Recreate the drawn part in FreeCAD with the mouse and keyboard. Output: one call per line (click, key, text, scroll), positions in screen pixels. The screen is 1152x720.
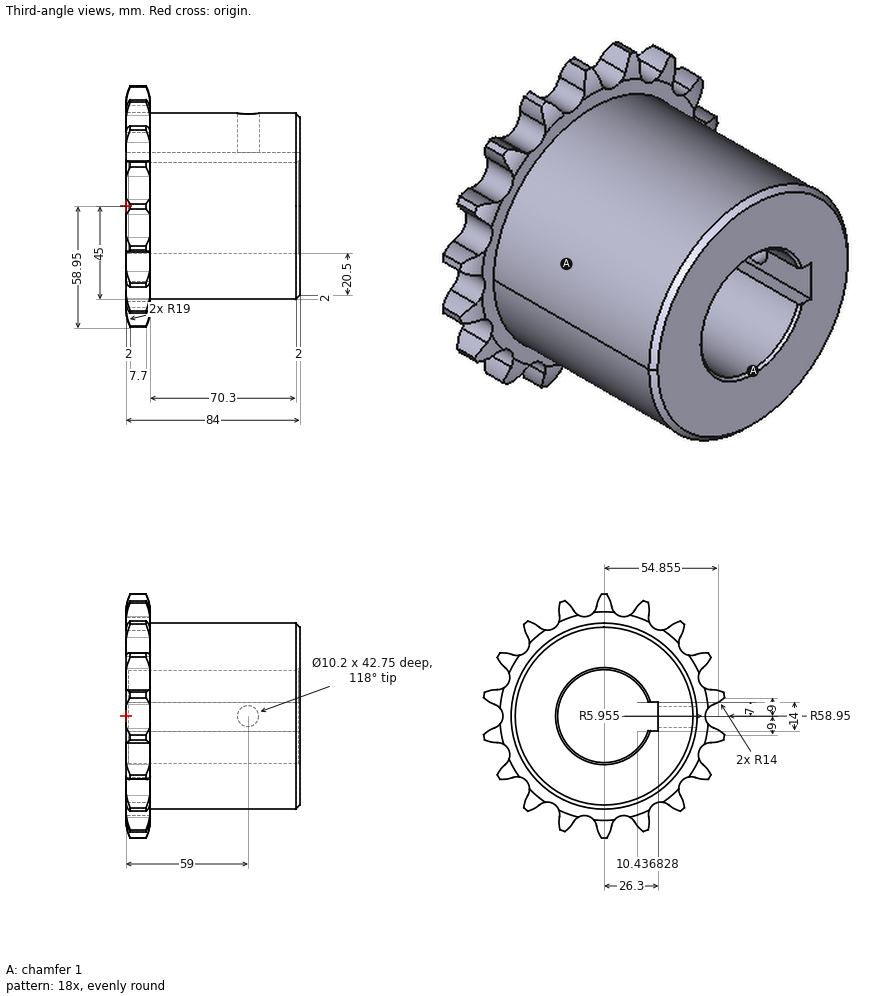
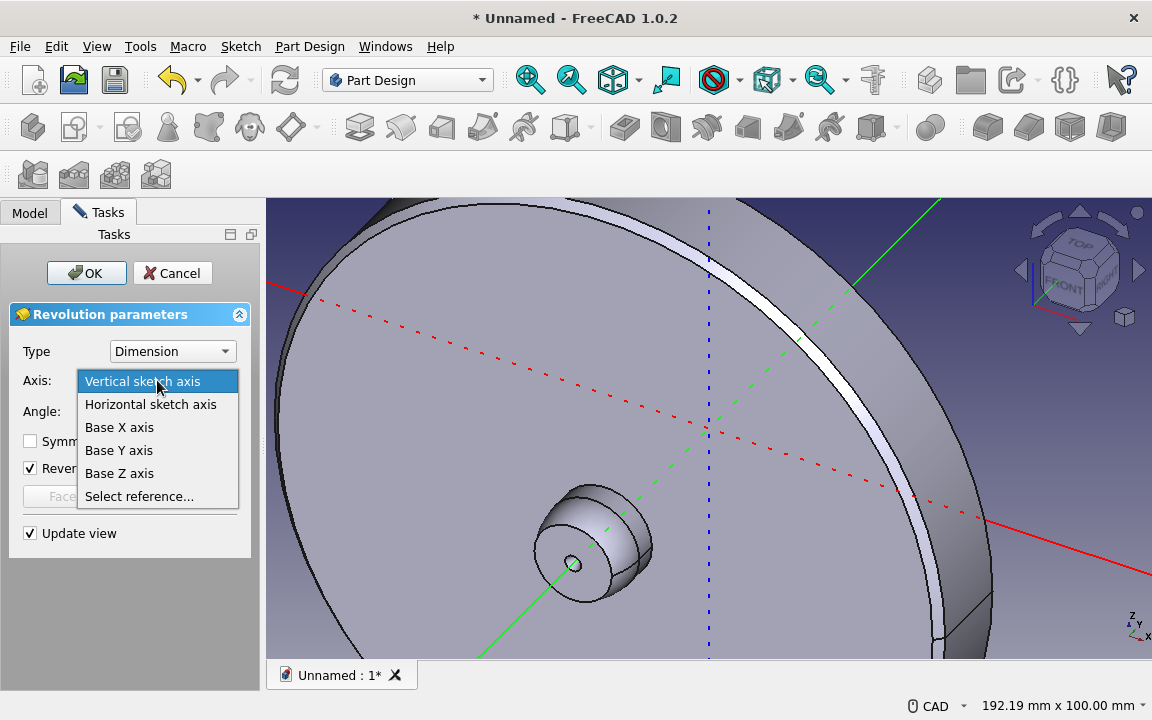
click(156, 404)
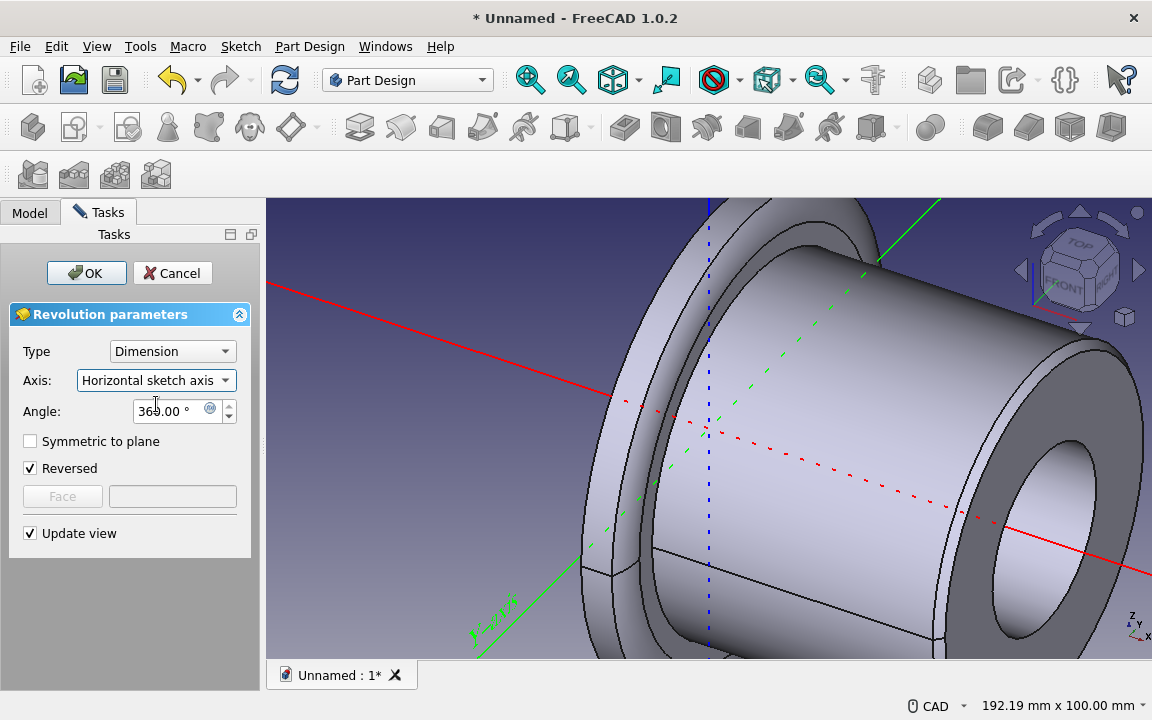
click(87, 273)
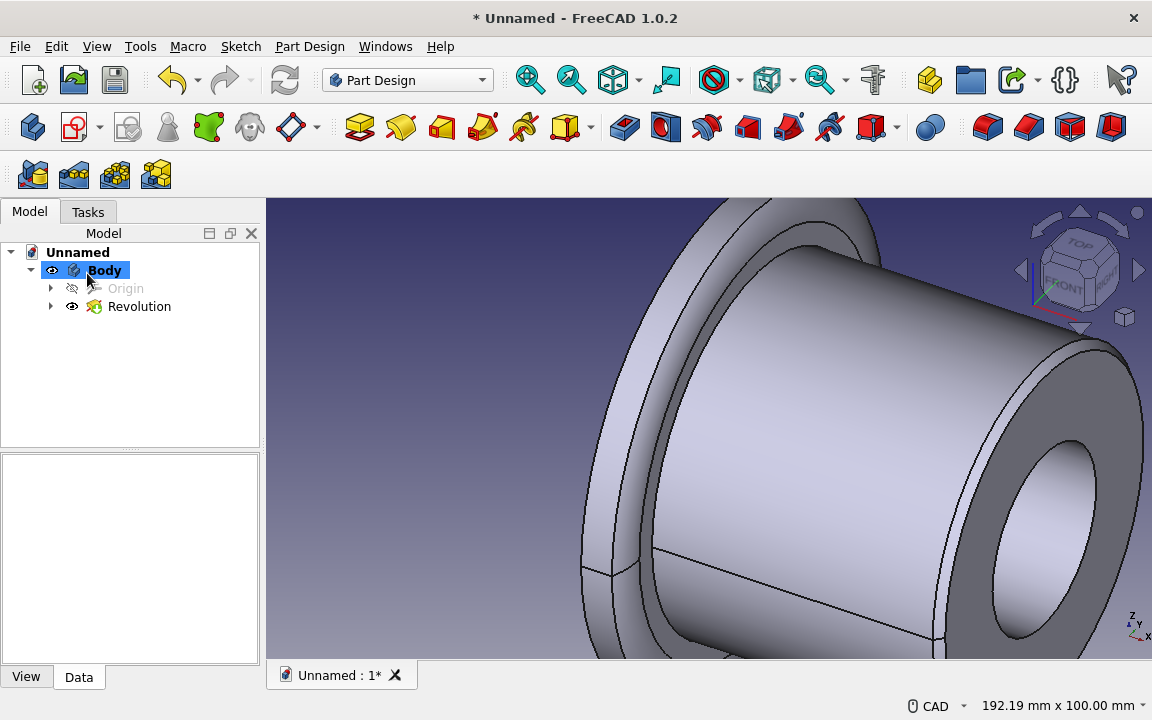
click(531, 80)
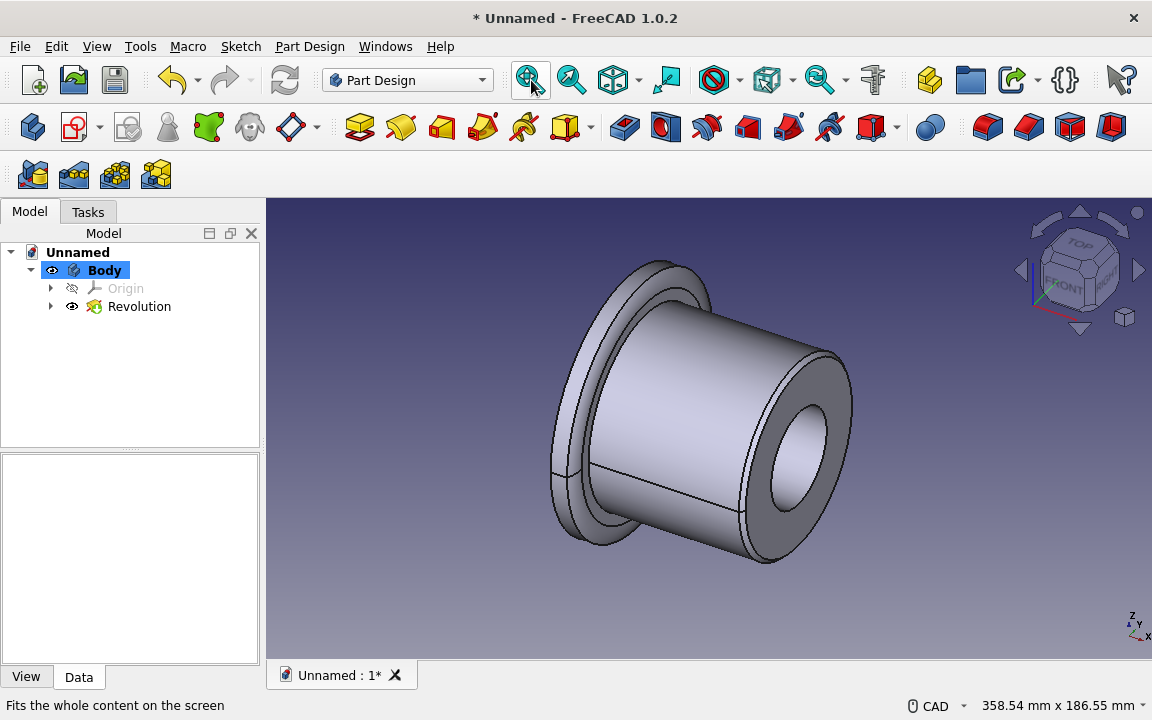
click(827, 430)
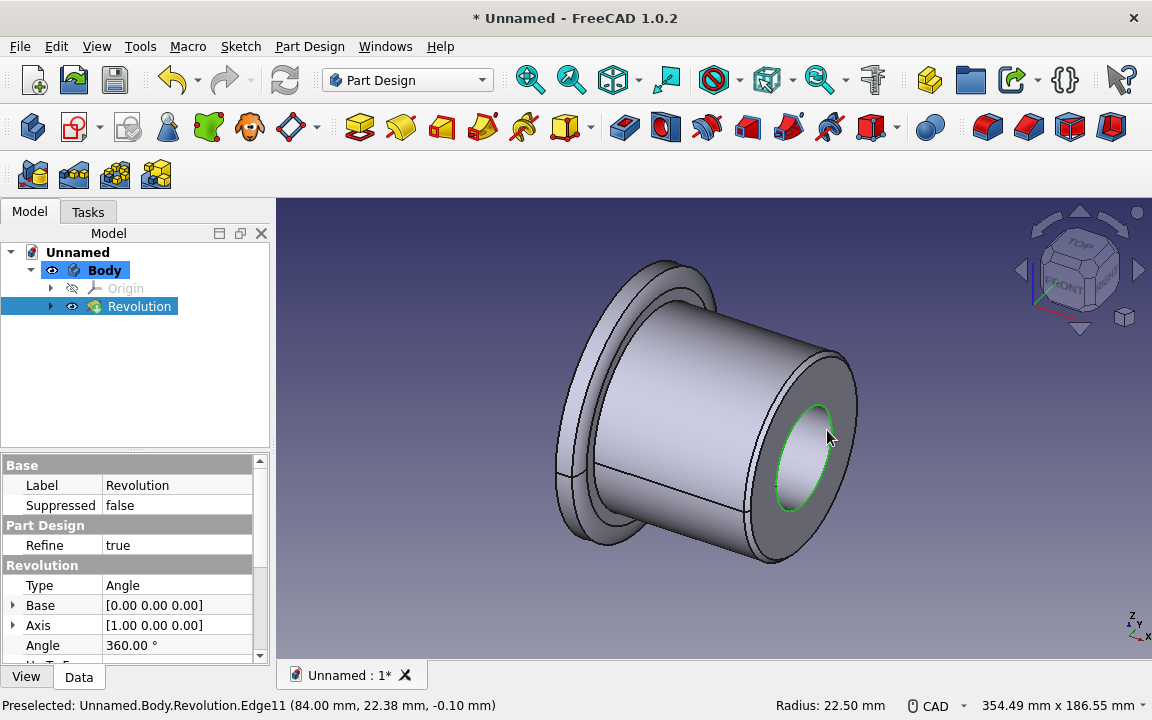
key(0)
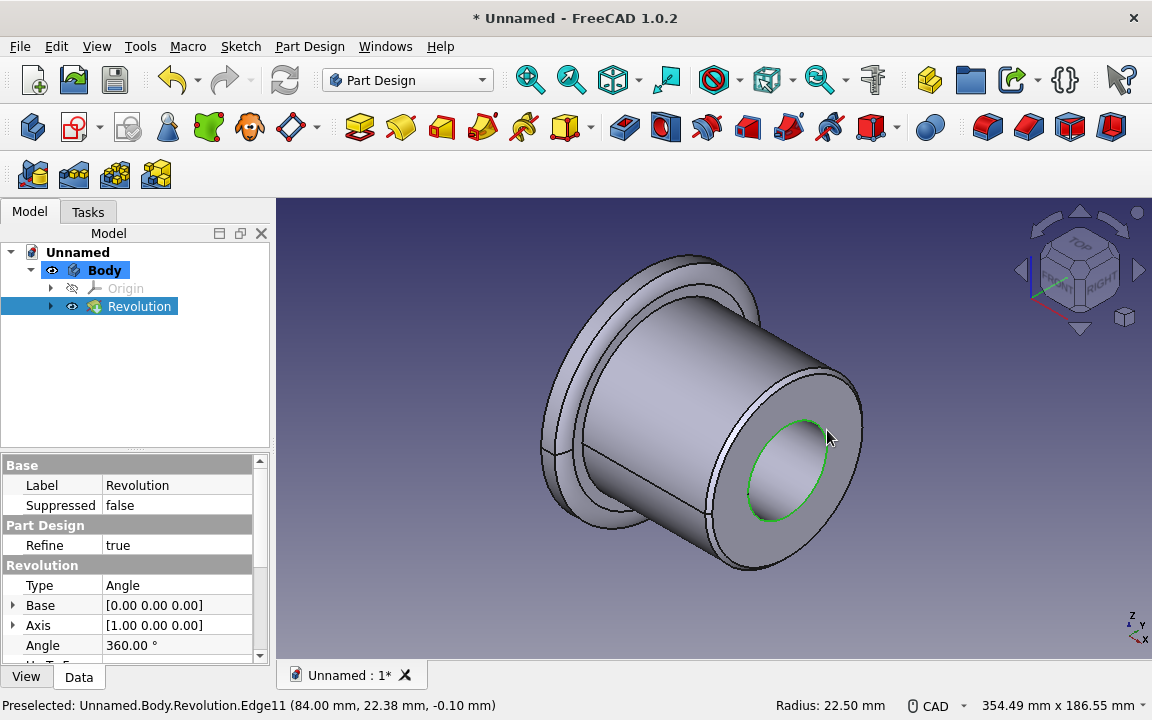
key(2)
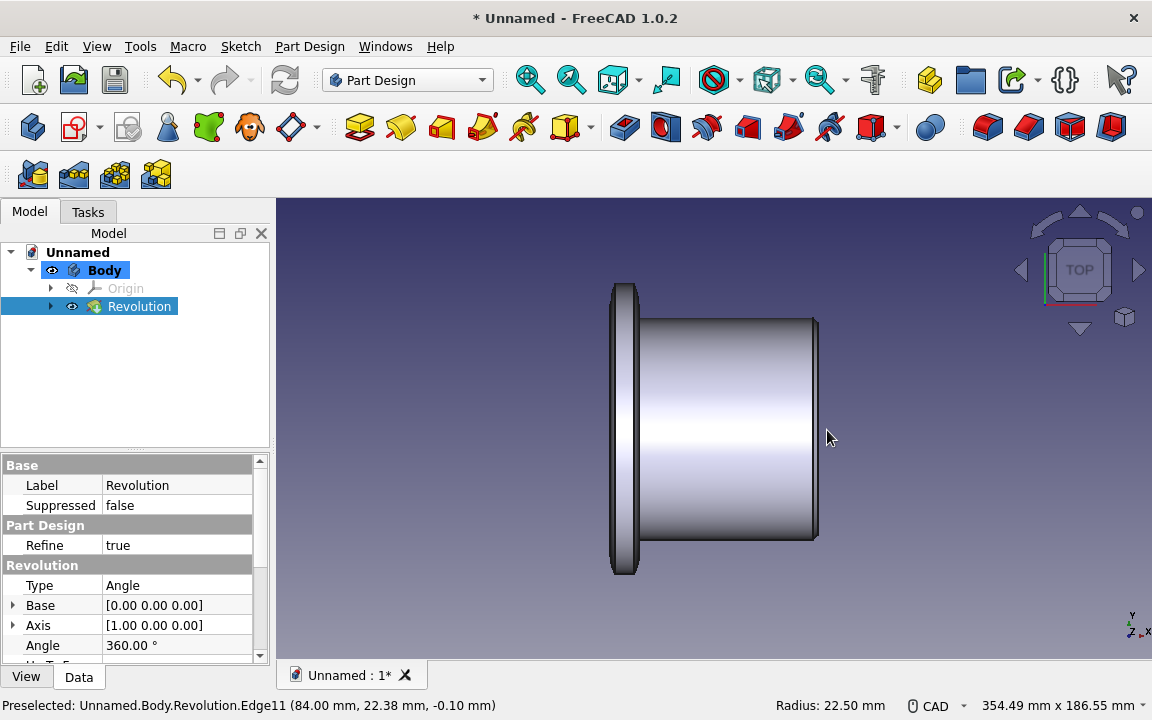
key(1)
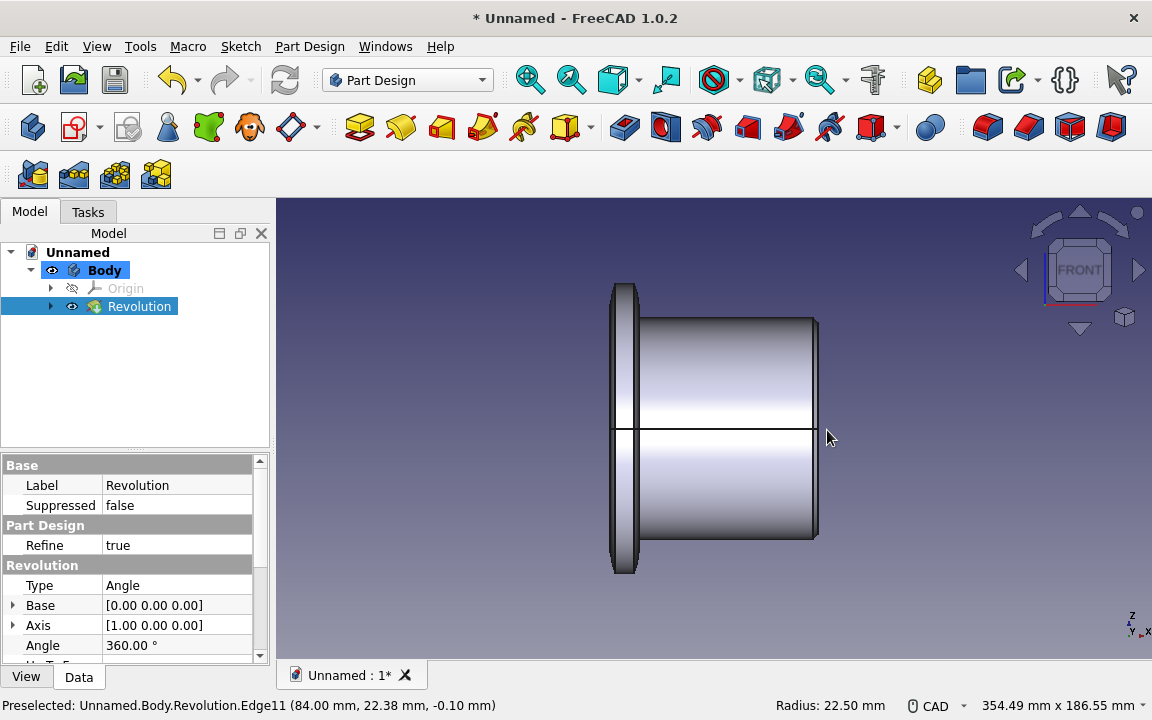
key(3)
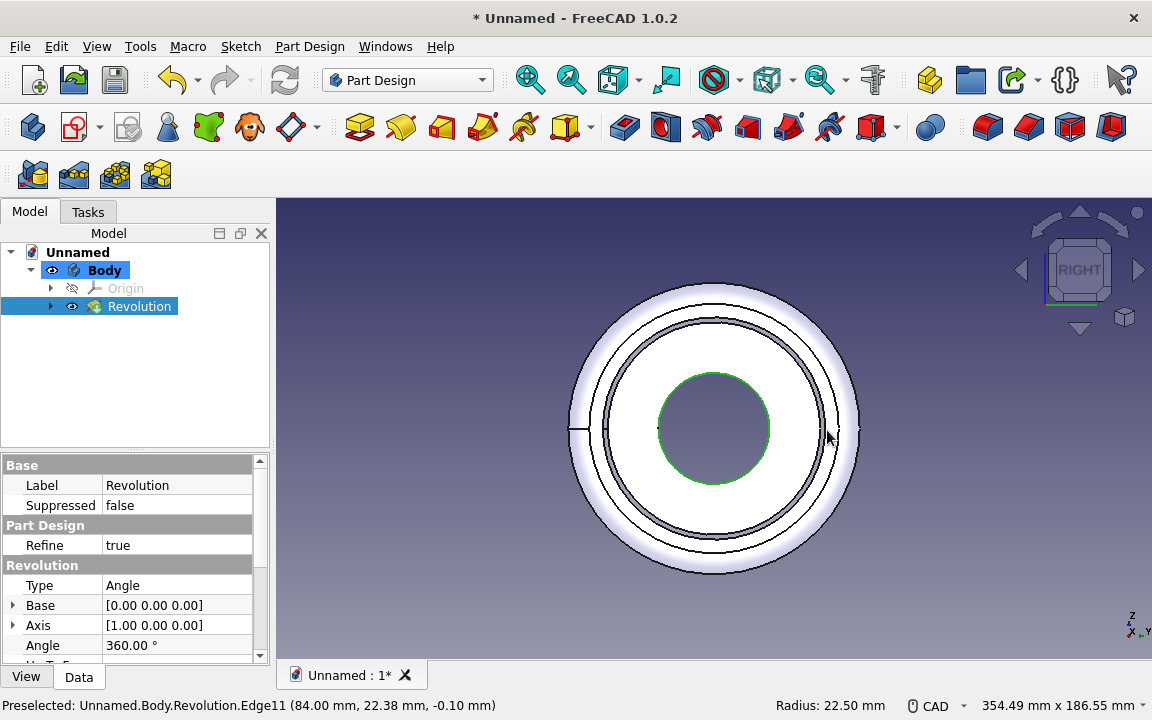
key(5)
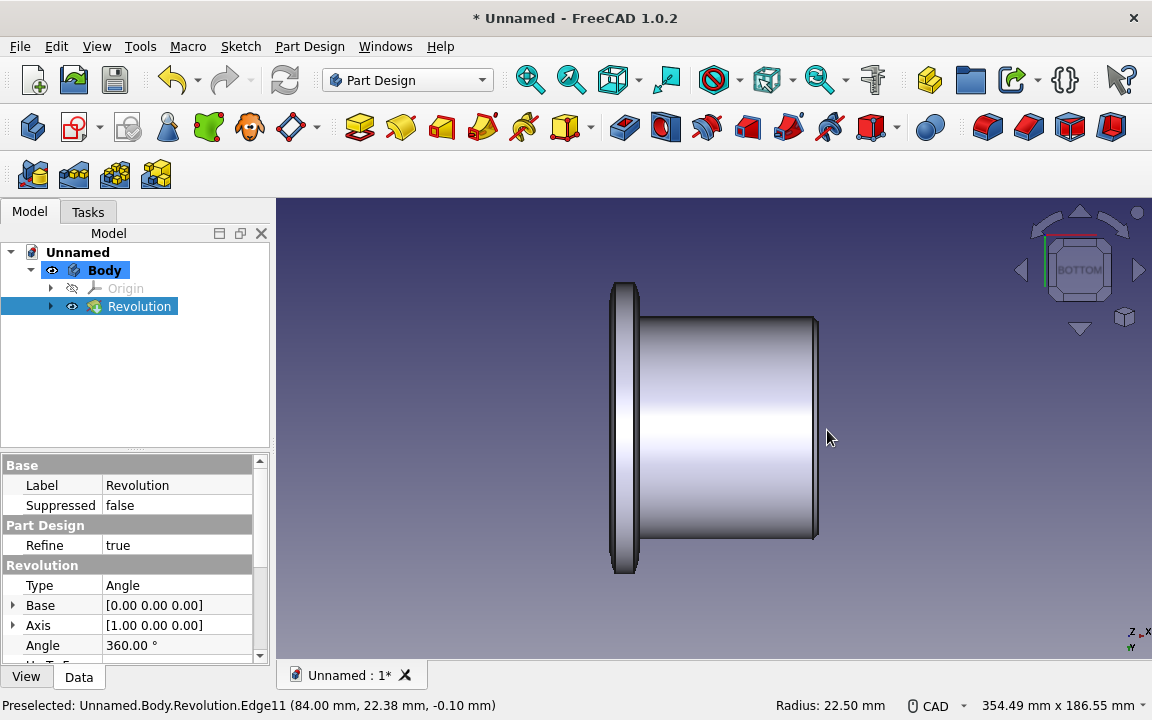
key(4)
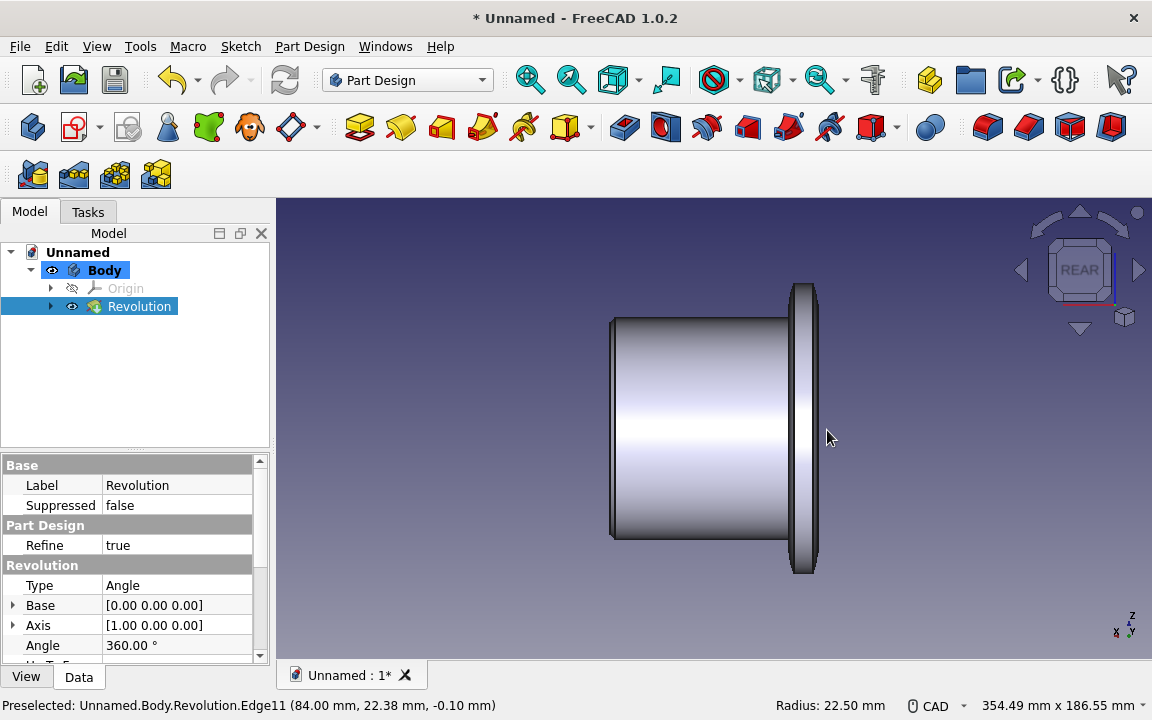
key(6)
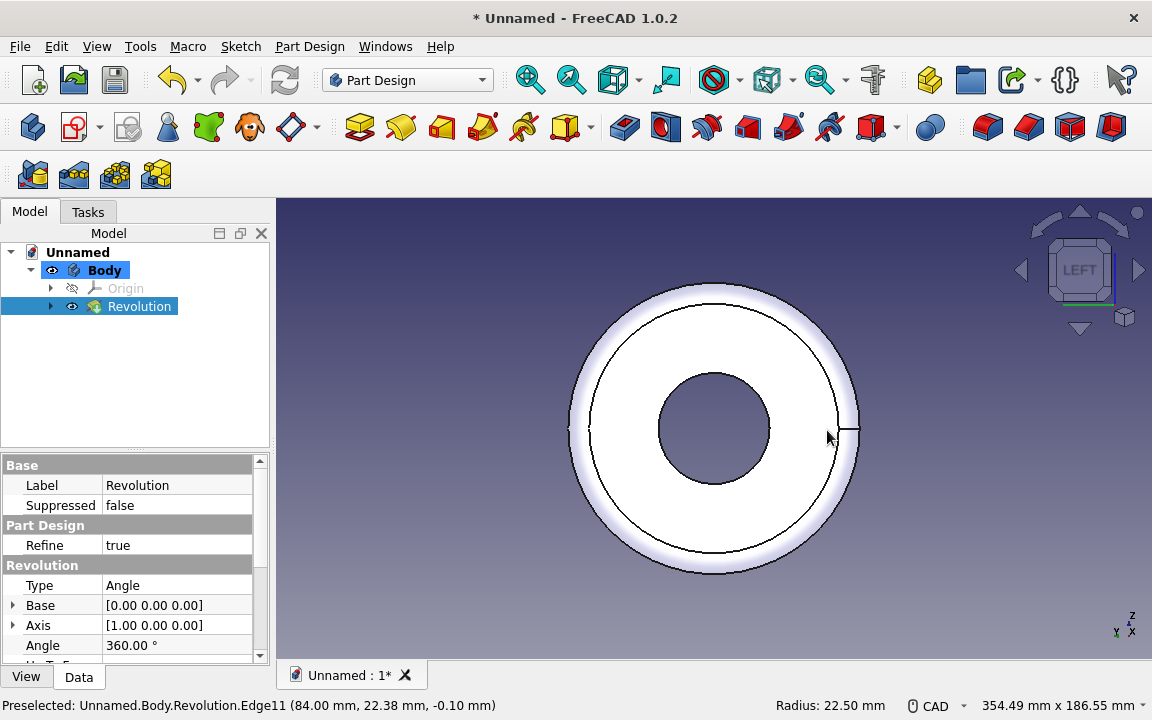
click(658, 427, ctrl)